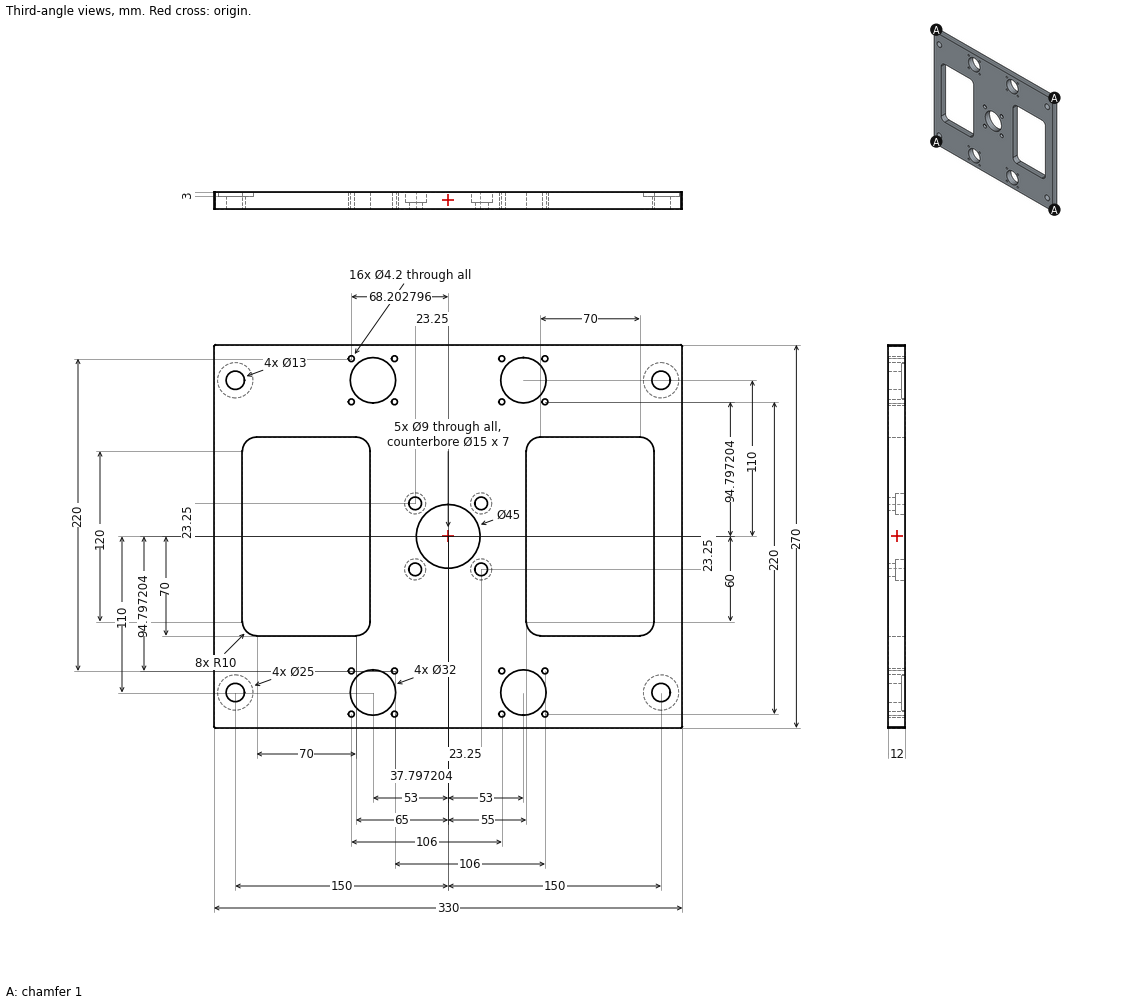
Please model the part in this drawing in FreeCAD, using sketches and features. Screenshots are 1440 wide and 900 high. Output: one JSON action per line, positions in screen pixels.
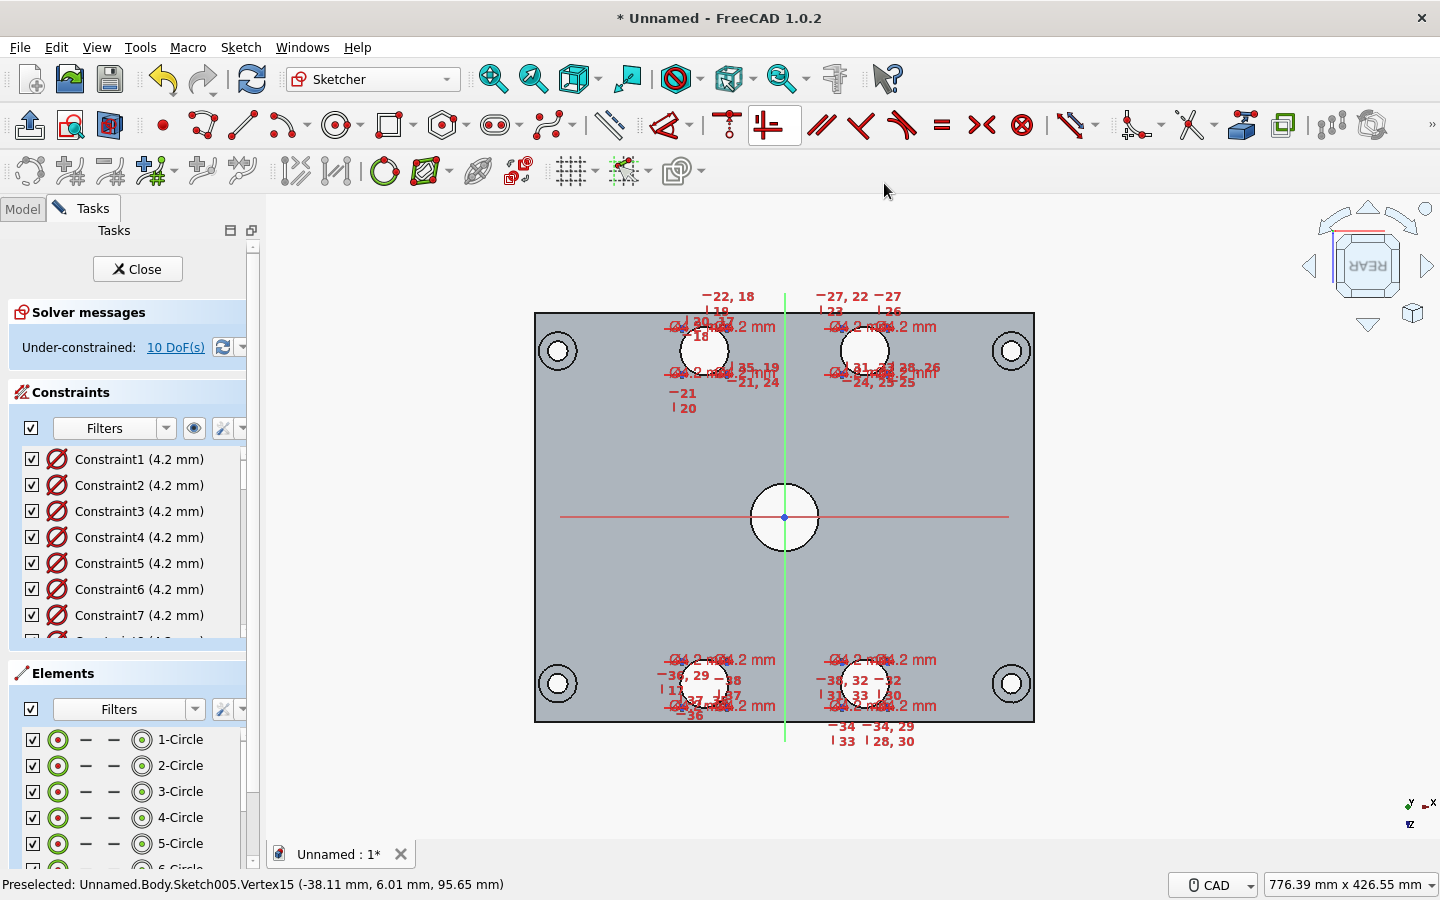
{"action": "left_click", "coordinate": [682, 708]}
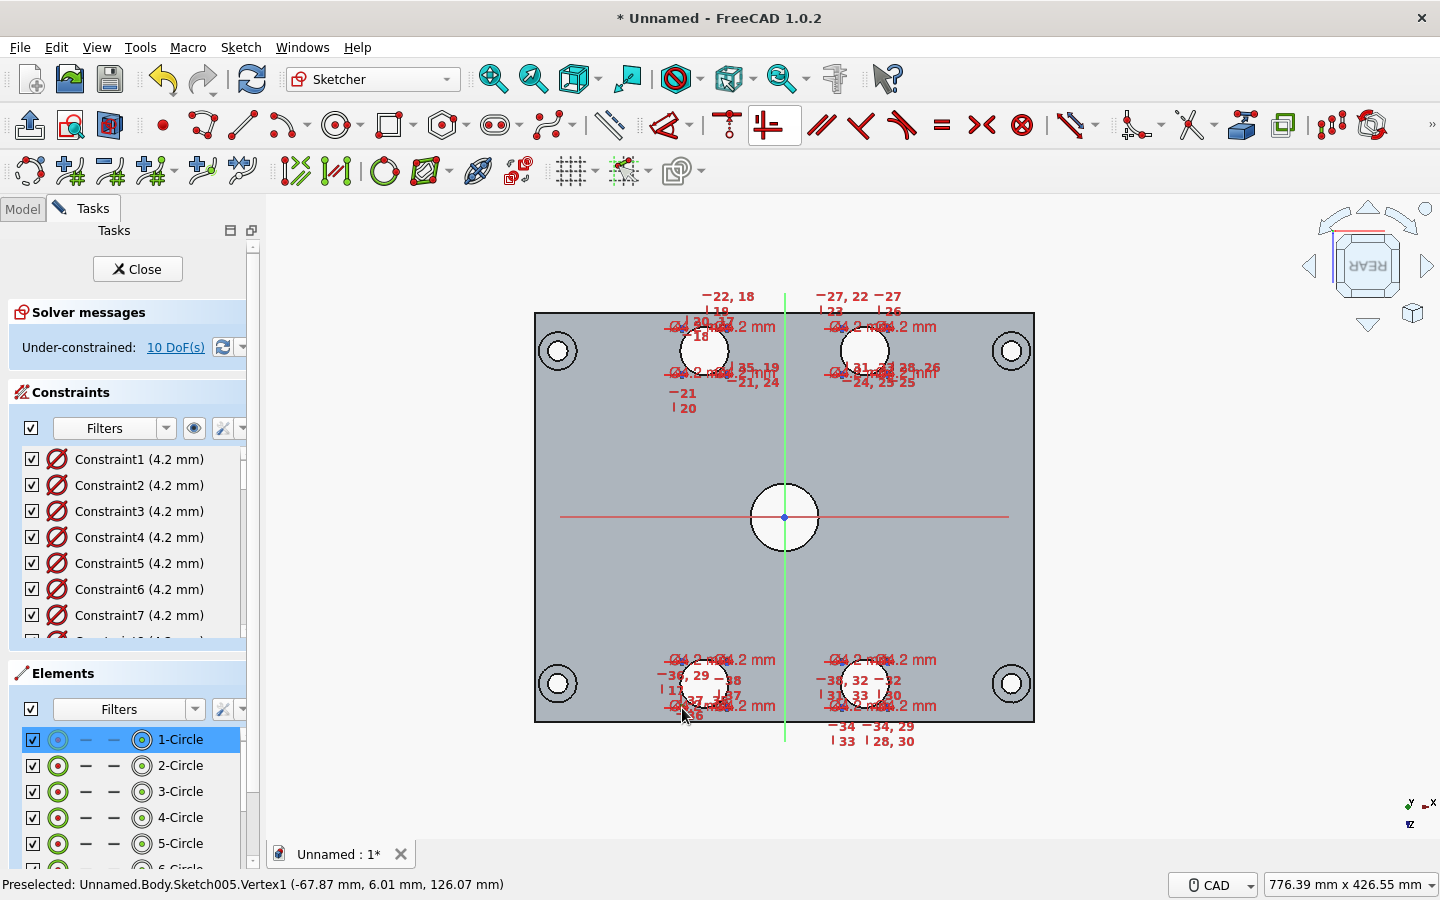
{"action": "left_click", "coordinate": [682, 662]}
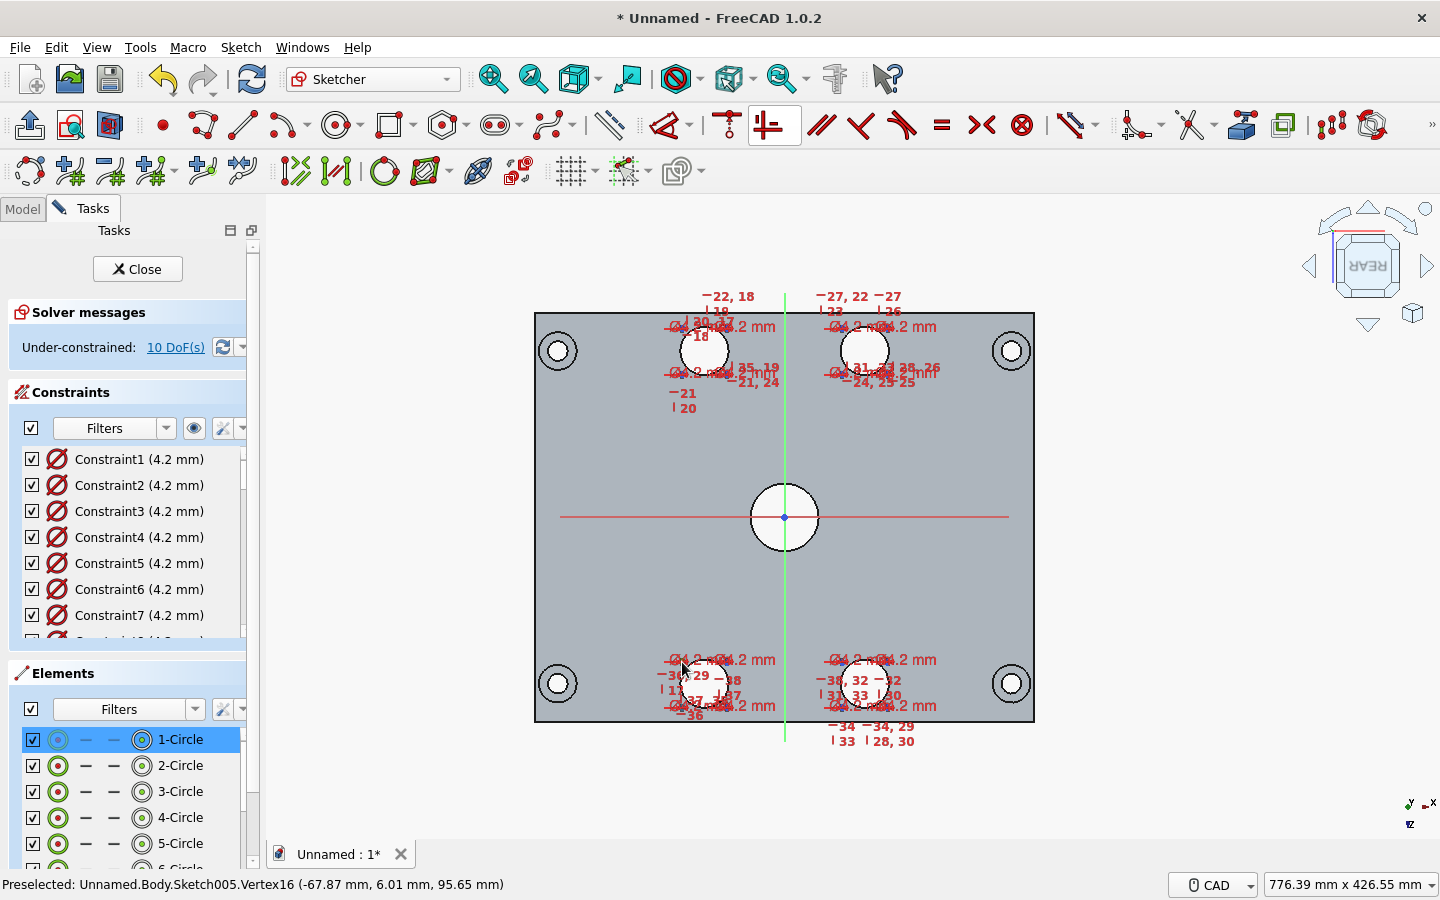
{"action": "left_click", "coordinate": [796, 126]}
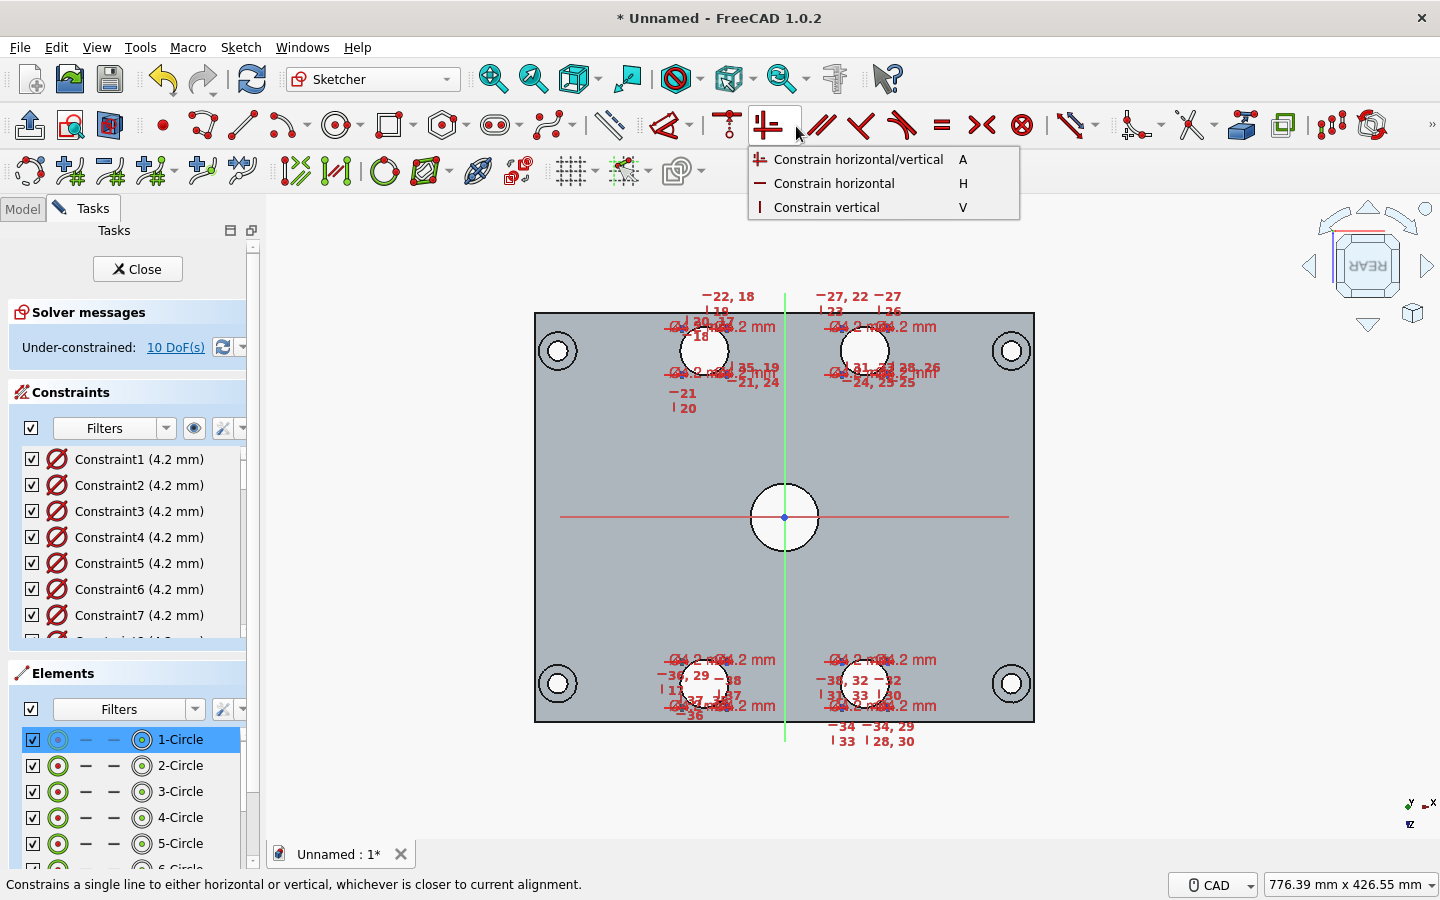
{"action": "left_click", "coordinate": [884, 207]}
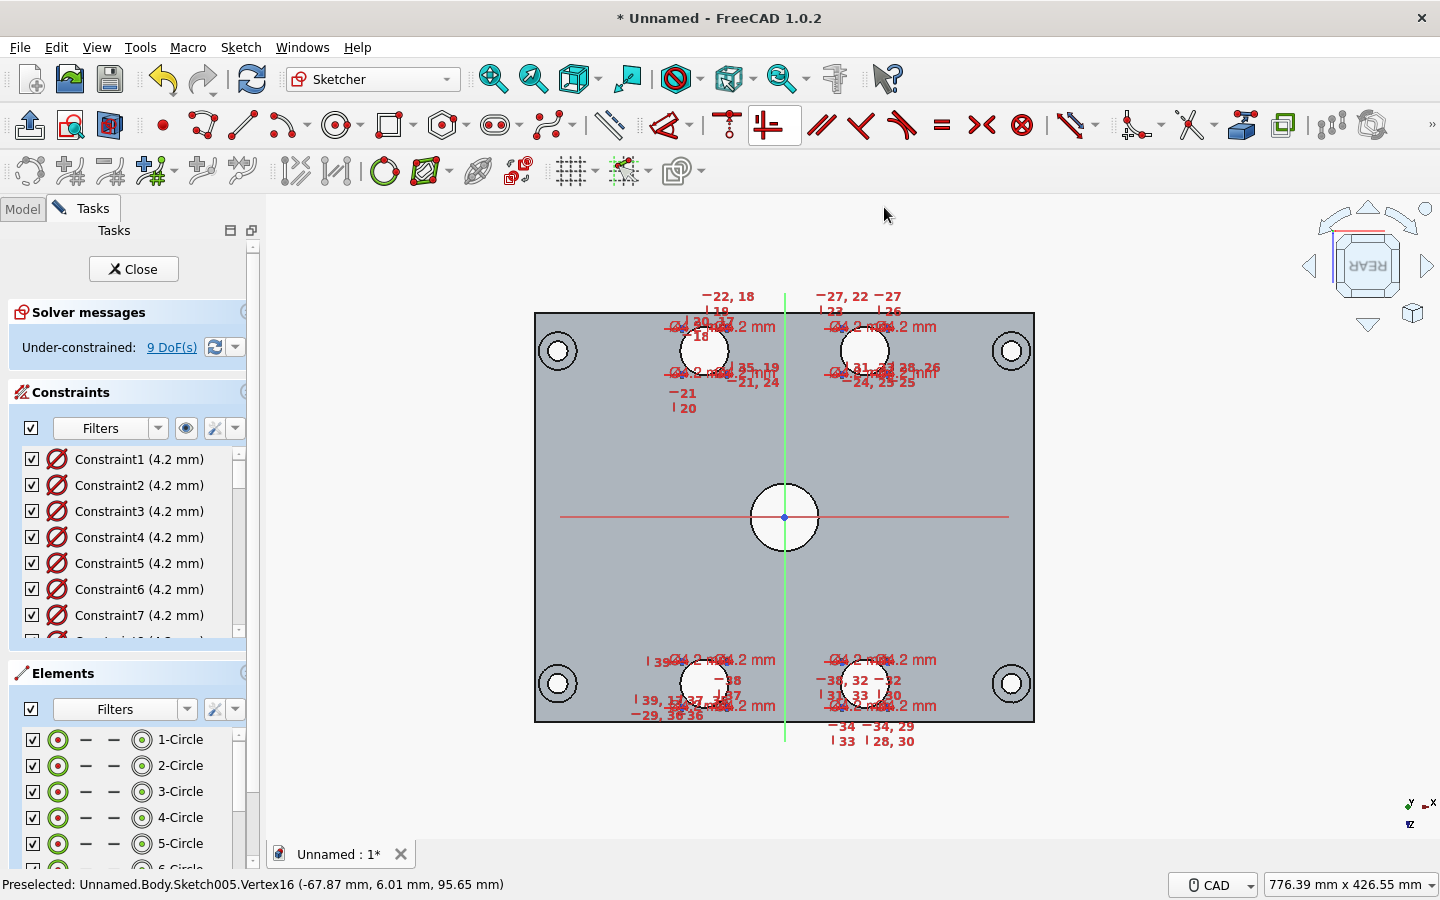
{"action": "left_click", "coordinate": [727, 662]}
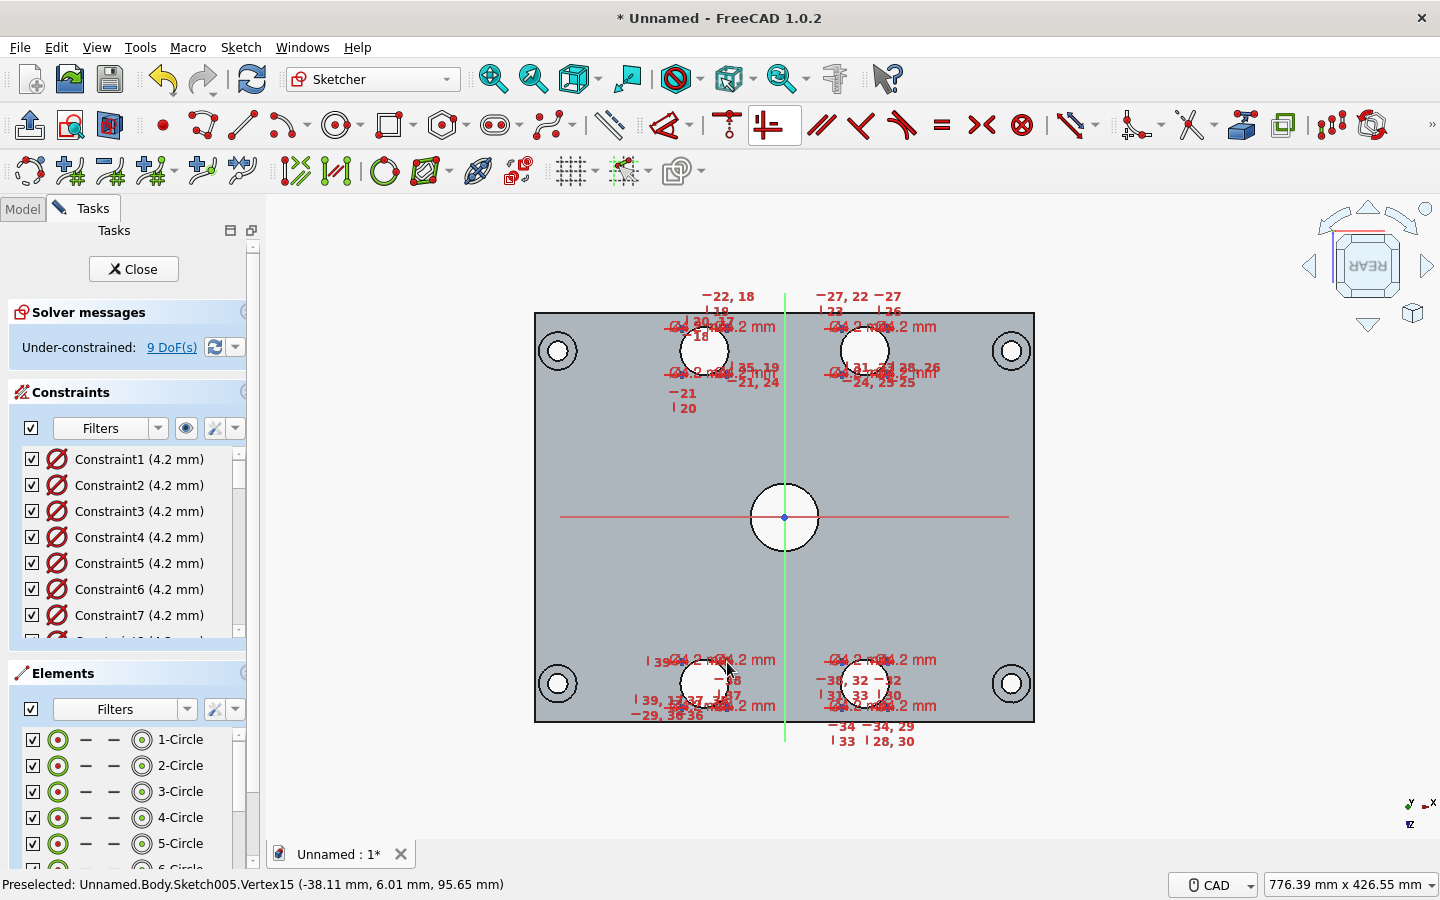
{"action": "left_click", "coordinate": [682, 662]}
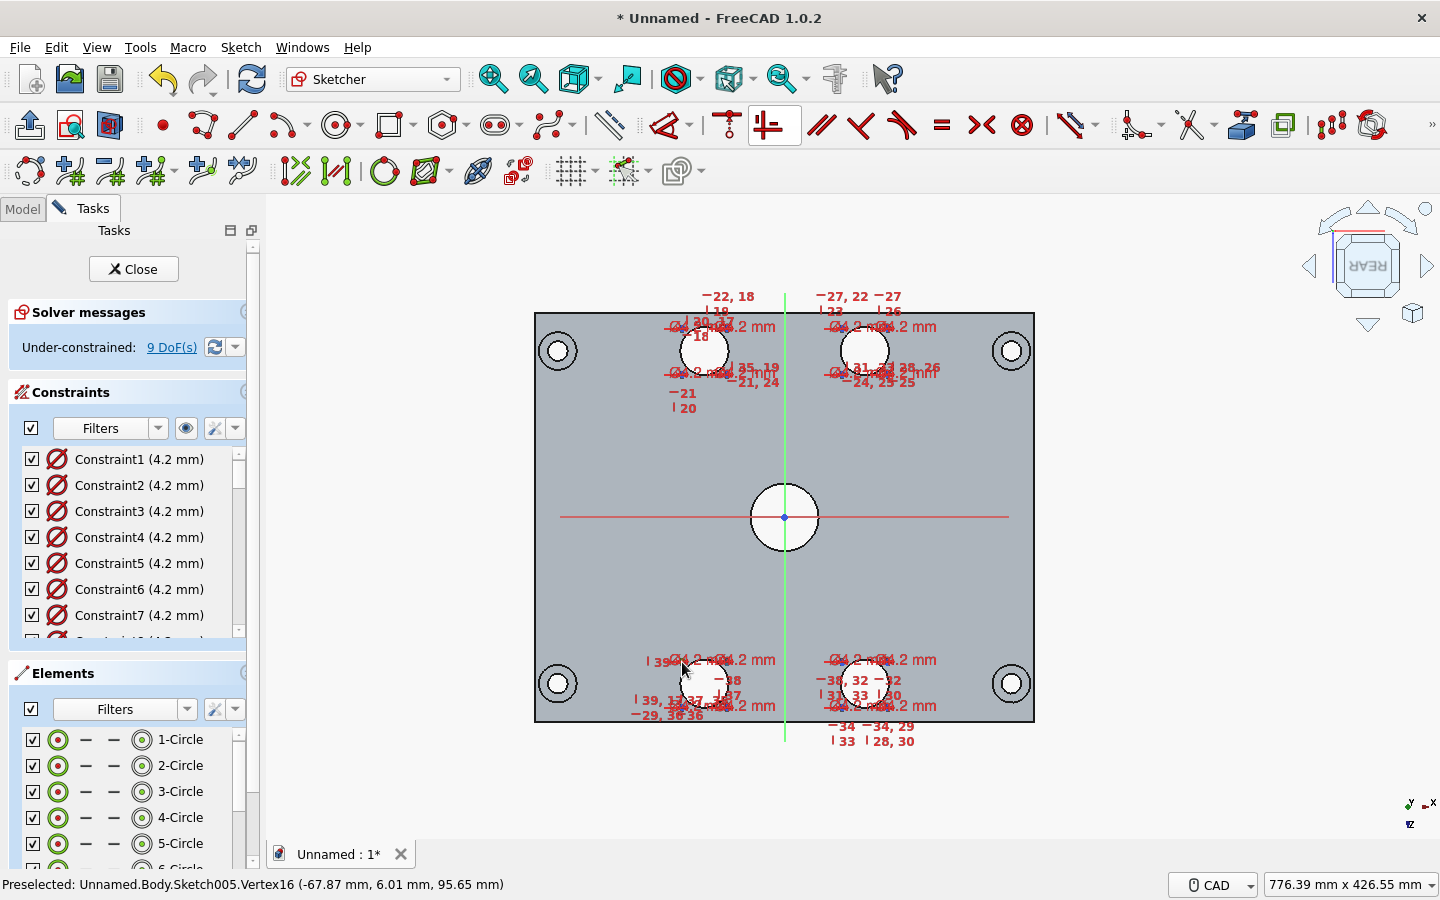
{"action": "key", "text": "h"}